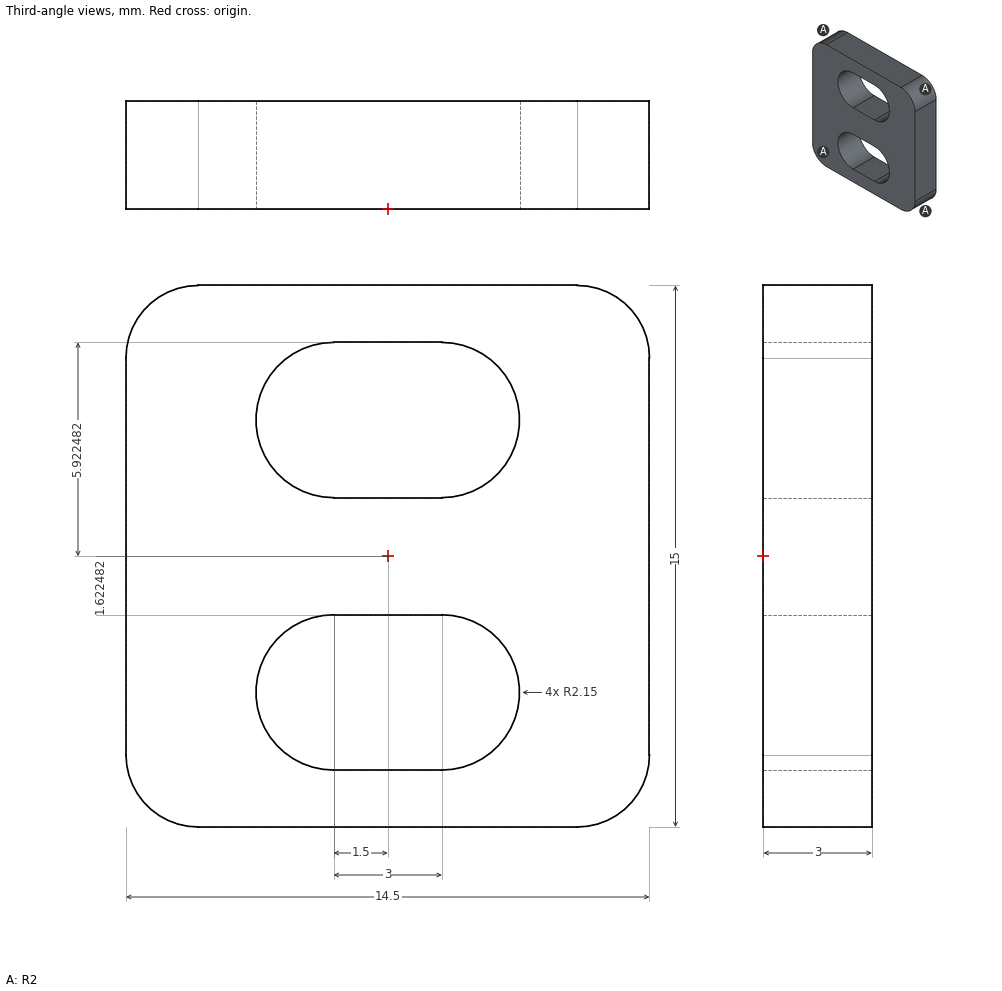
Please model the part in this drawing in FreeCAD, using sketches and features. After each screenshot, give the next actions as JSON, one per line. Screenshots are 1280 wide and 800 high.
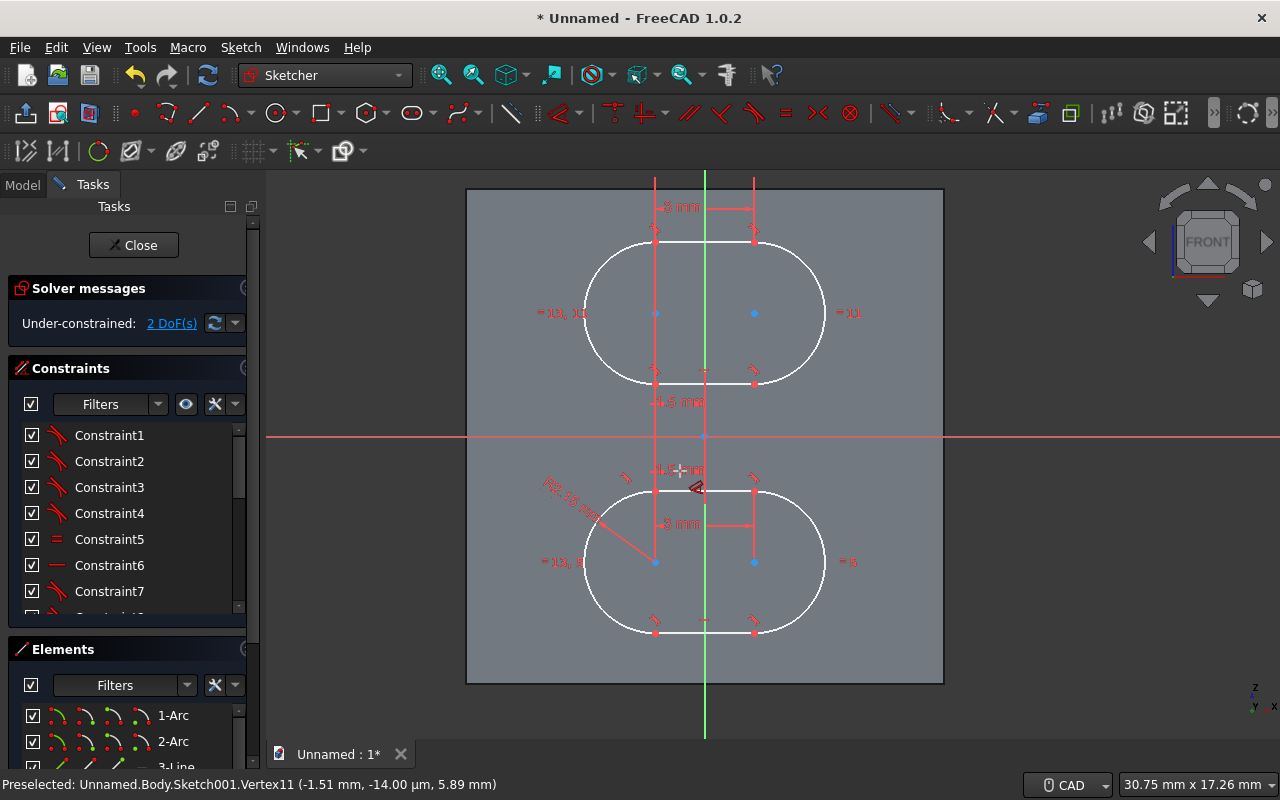
{"action": "left_click", "coordinate": [655, 491]}
{"action": "left_click", "coordinate": [597, 464]}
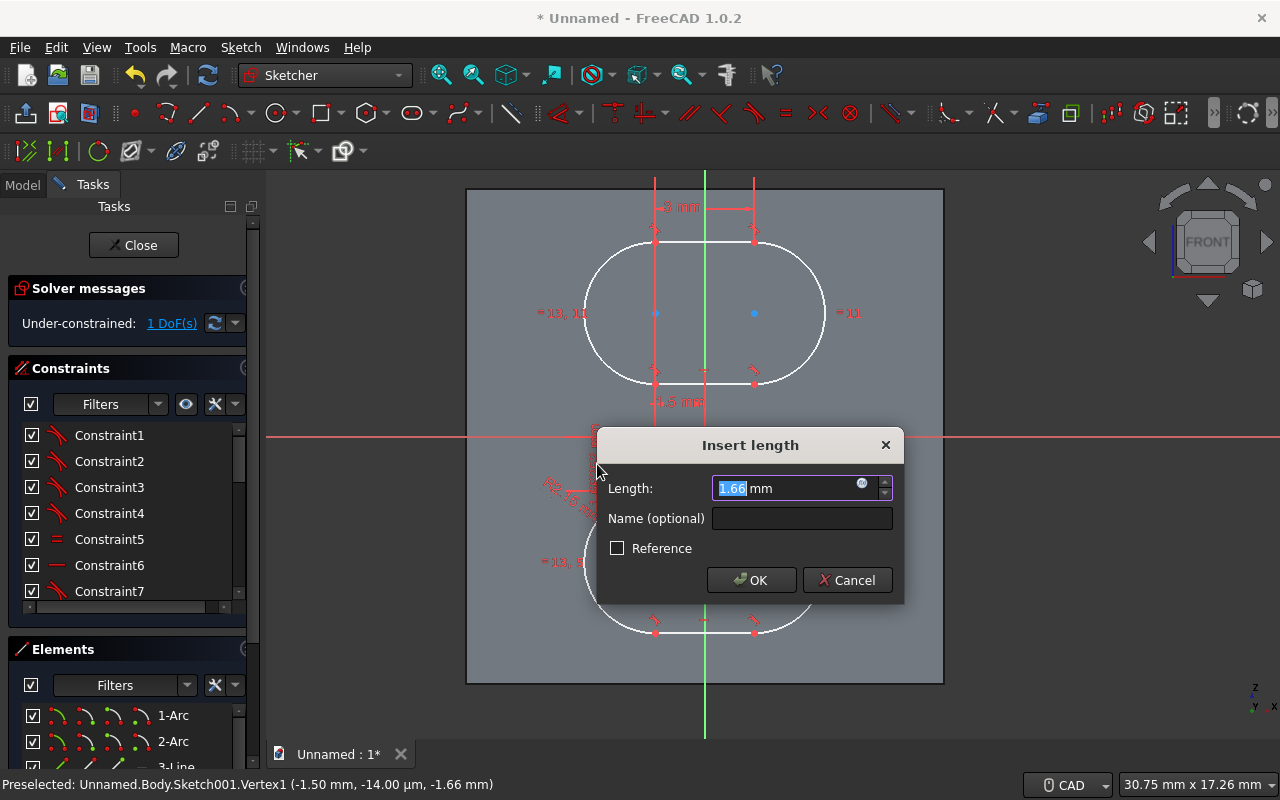
{"action": "type", "text": "1.622482"}
{"action": "key", "text": "Return"}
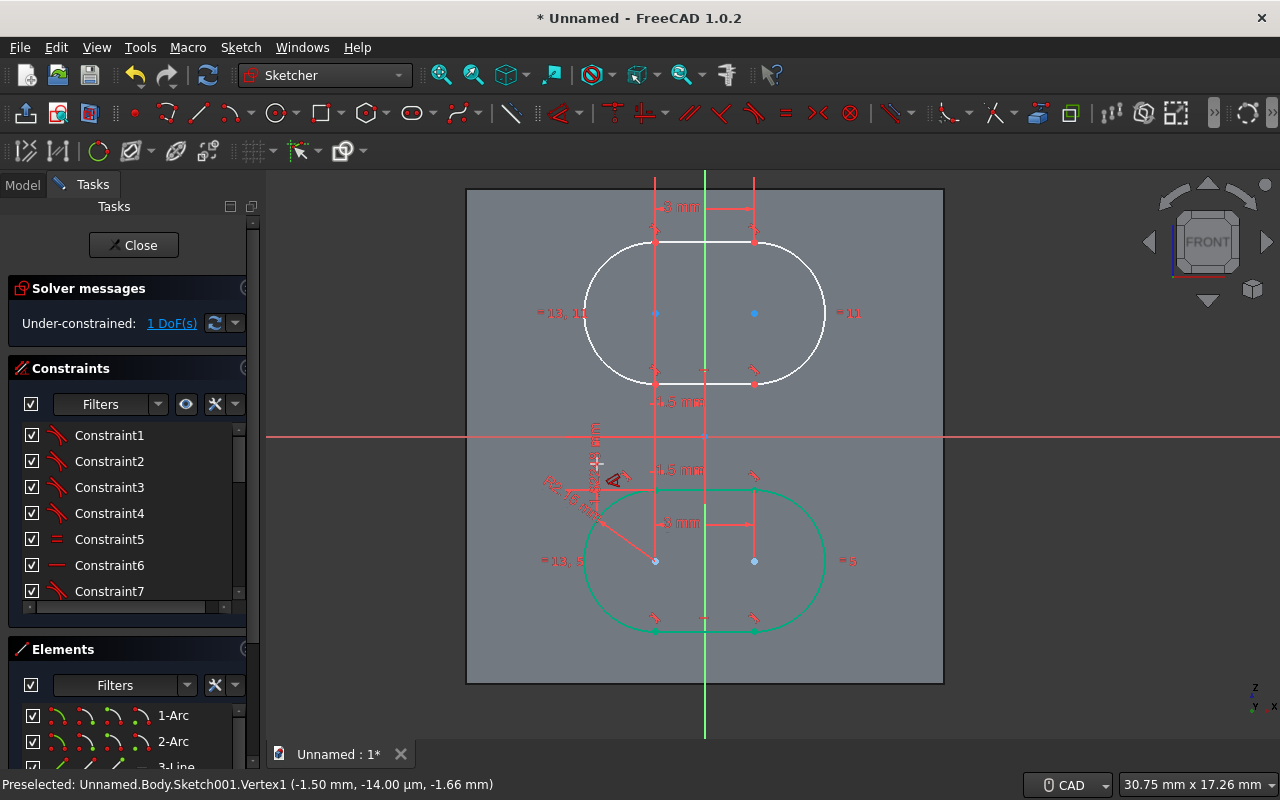
{"action": "left_click", "coordinate": [655, 242]}
{"action": "left_click", "coordinate": [621, 340]}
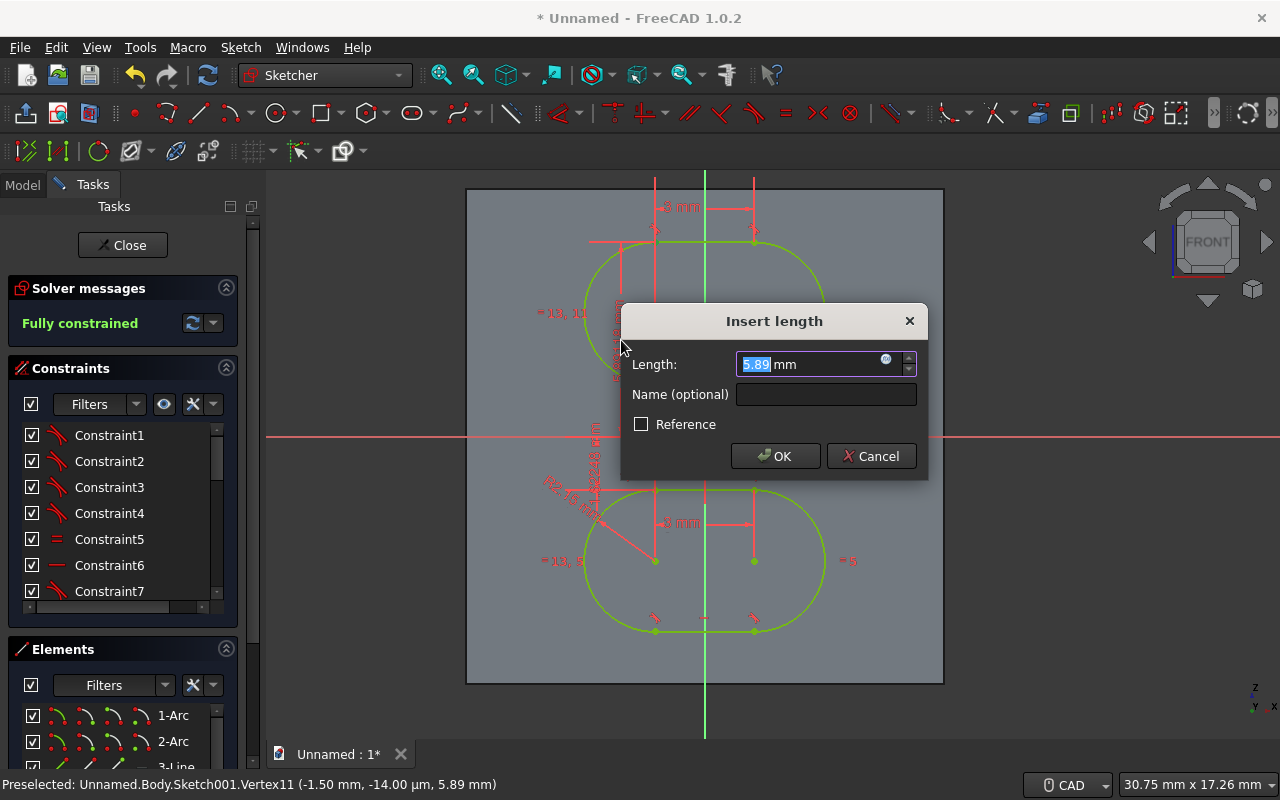
{"action": "type", "text": "5.922482"}
{"action": "key", "text": "Return"}
{"action": "key", "text": "Escape"}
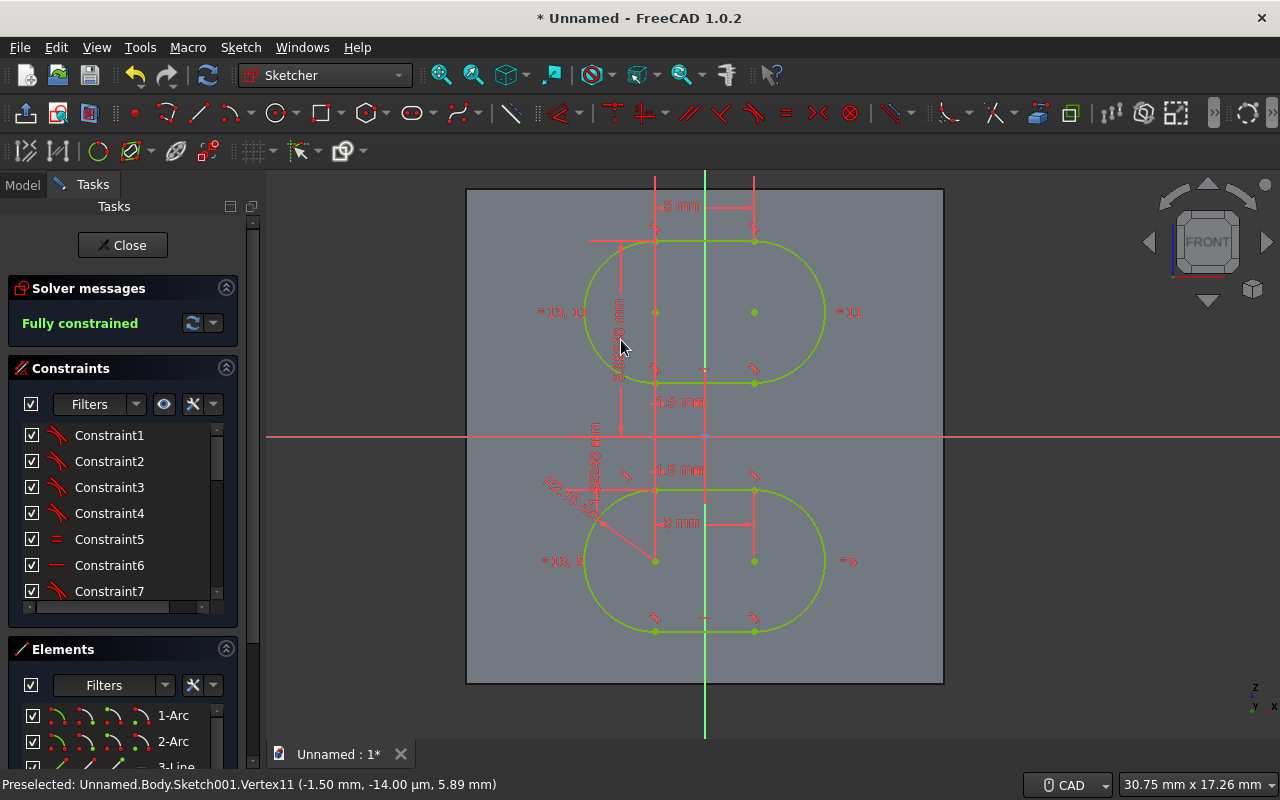
{"action": "left_click", "coordinate": [123, 245]}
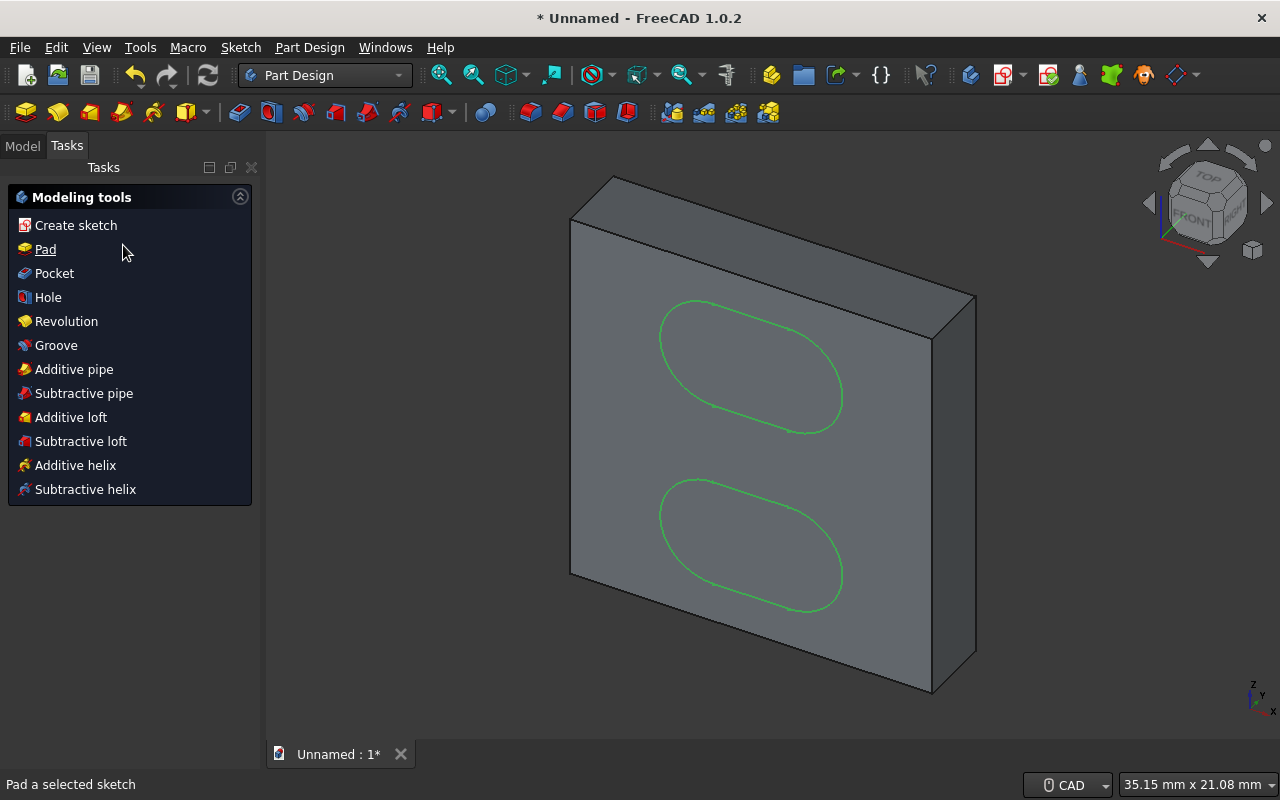
{"action": "left_click", "coordinate": [240, 112]}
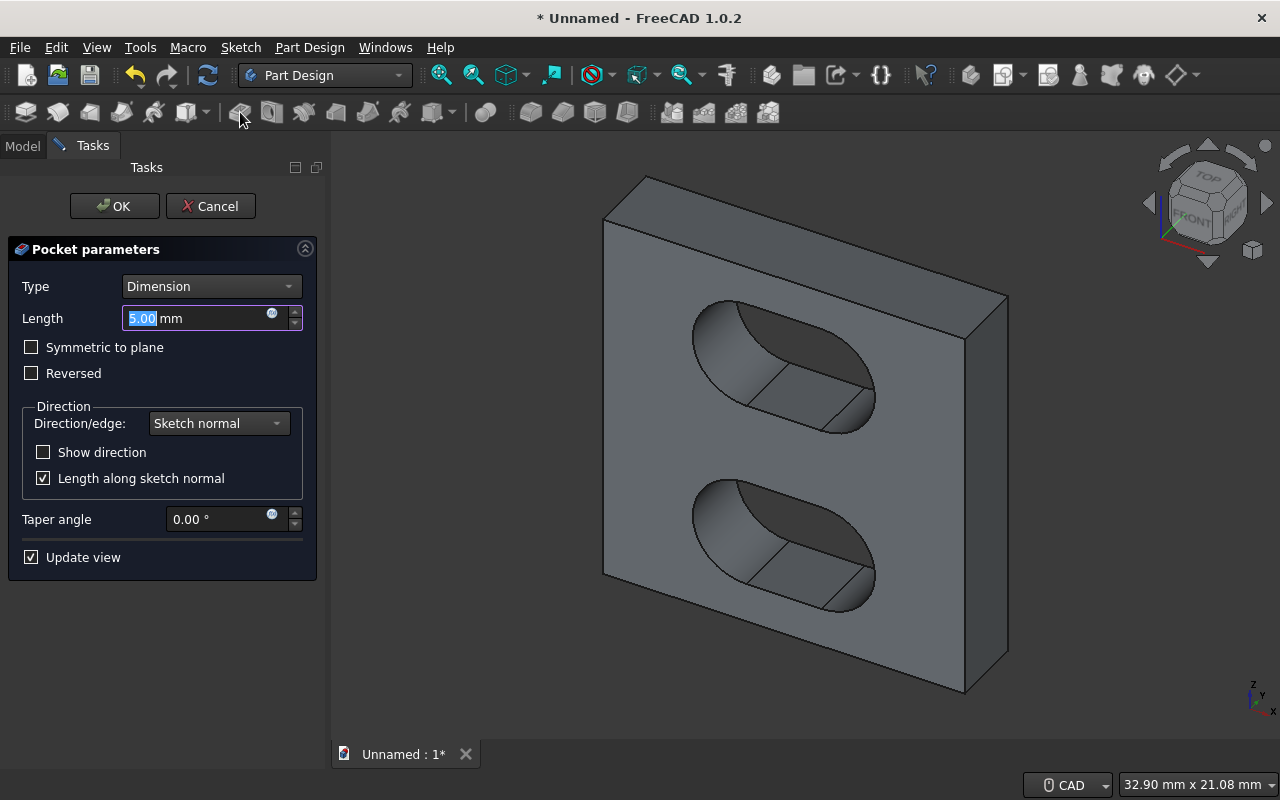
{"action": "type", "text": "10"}
{"action": "key", "text": "Tab"}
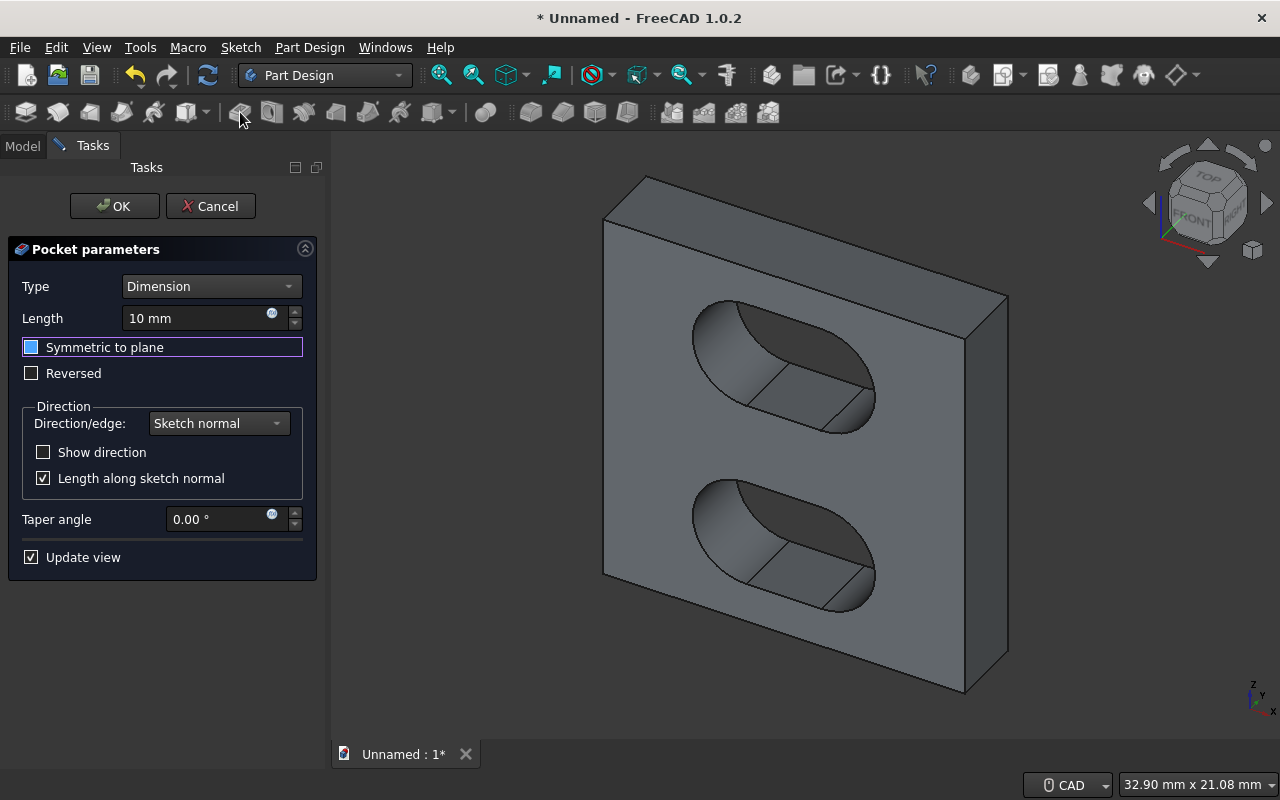
{"action": "left_click", "coordinate": [115, 206]}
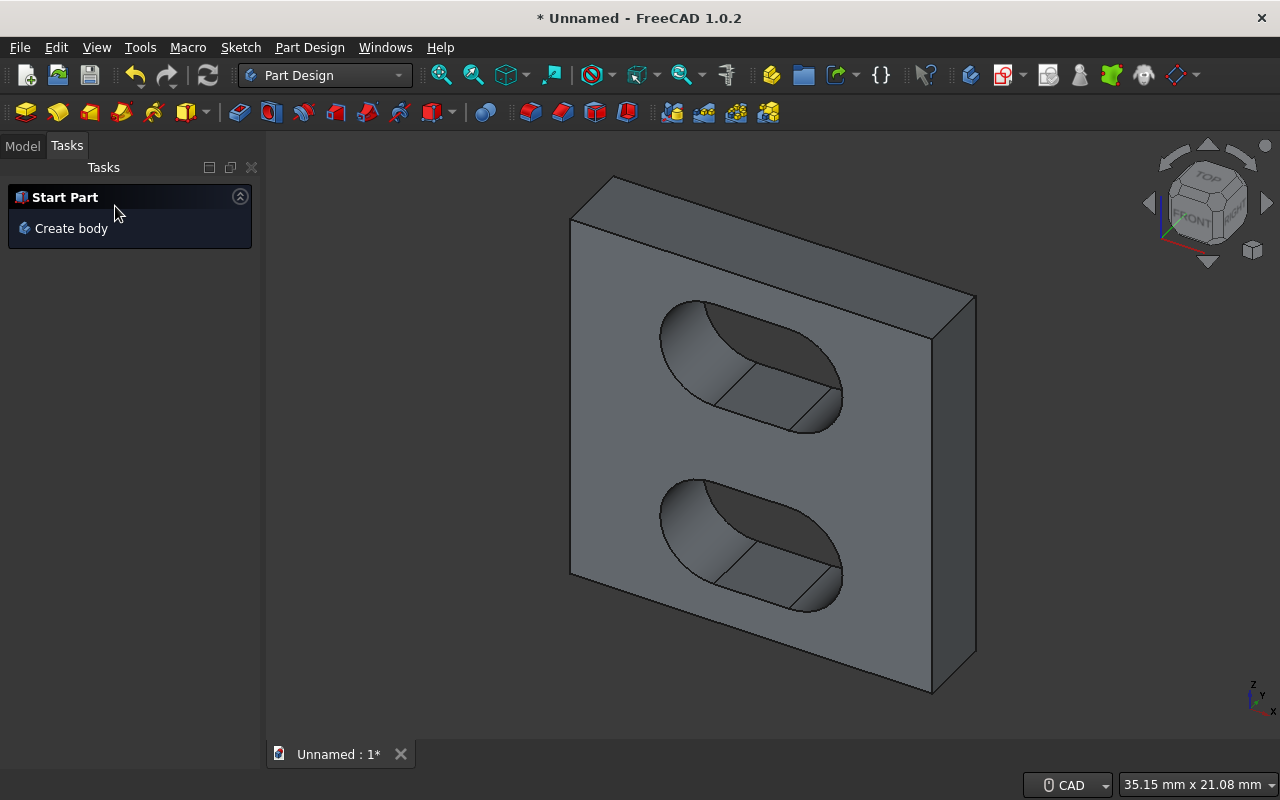
{"action": "left_click", "coordinate": [954, 317]}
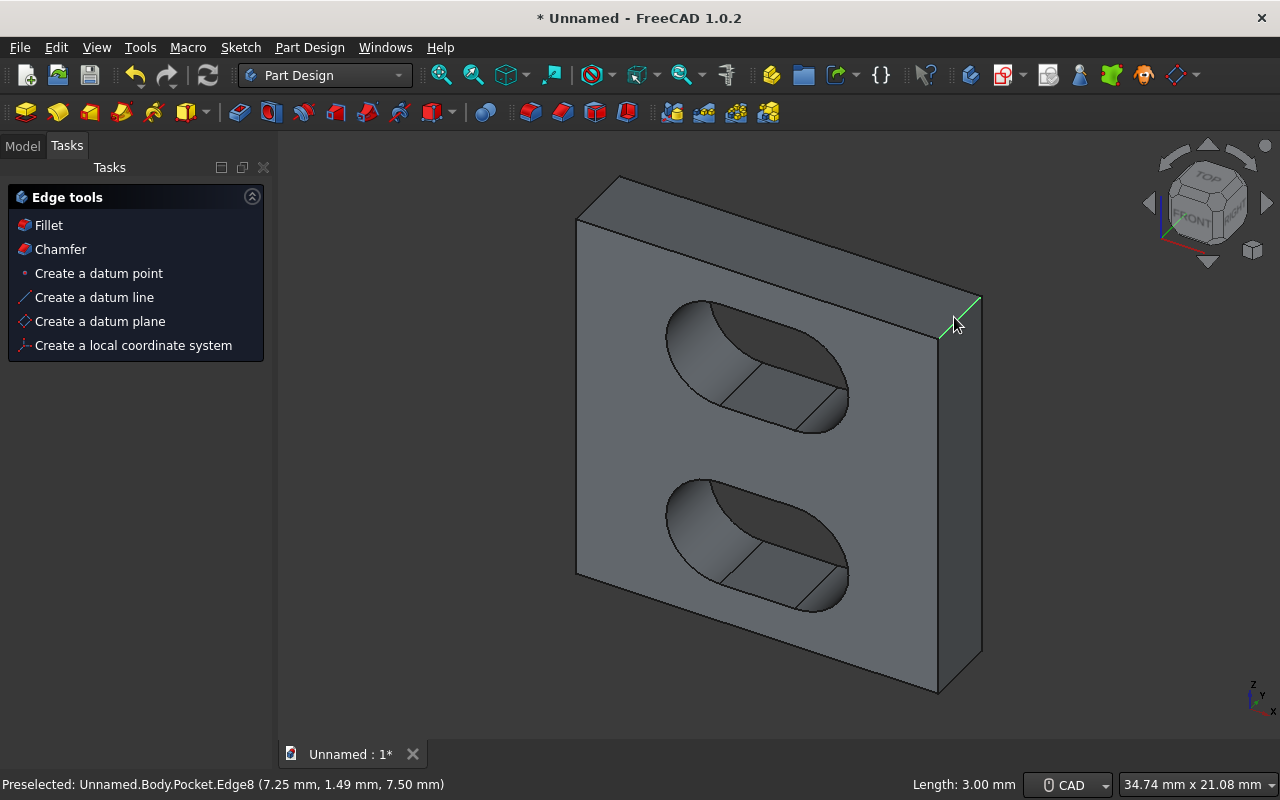
{"action": "key", "text": "0"}